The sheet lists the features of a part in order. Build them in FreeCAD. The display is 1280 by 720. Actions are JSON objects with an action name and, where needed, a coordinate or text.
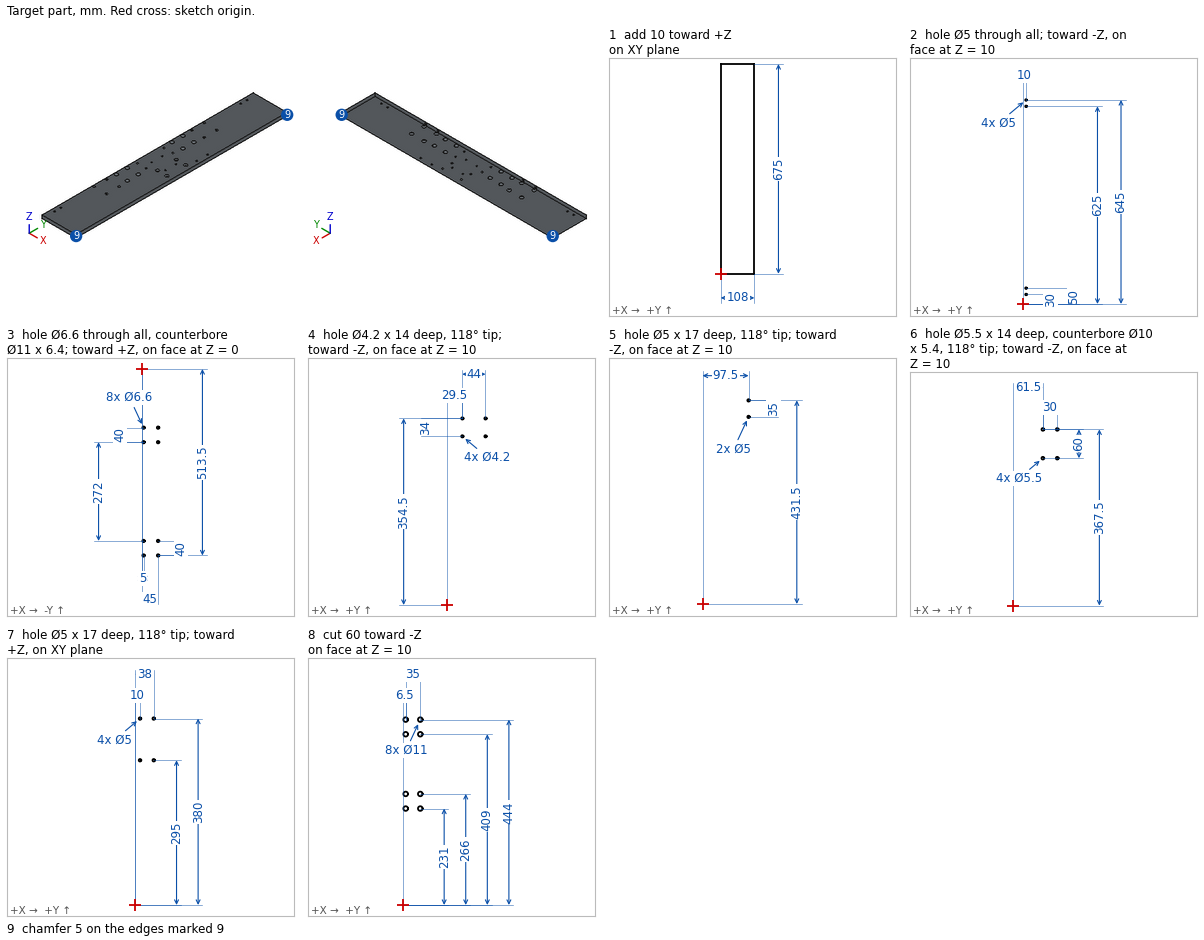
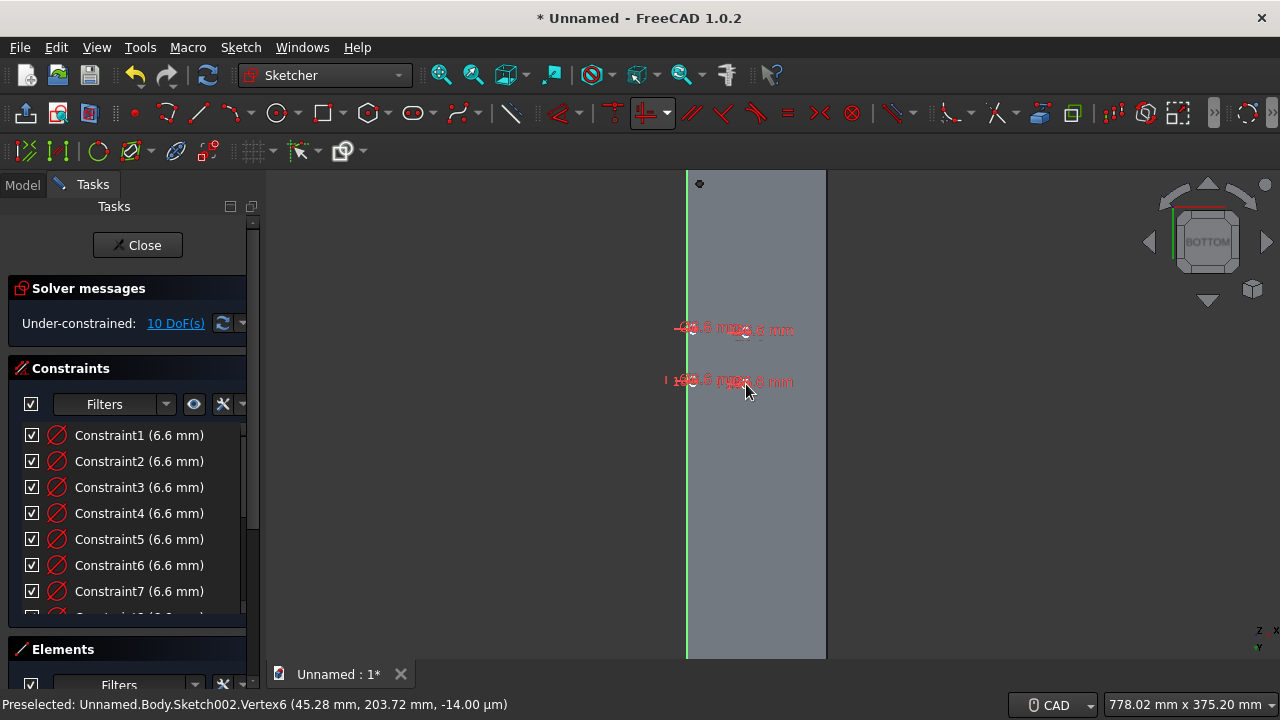
{"action": "left_click", "coordinate": [670, 114]}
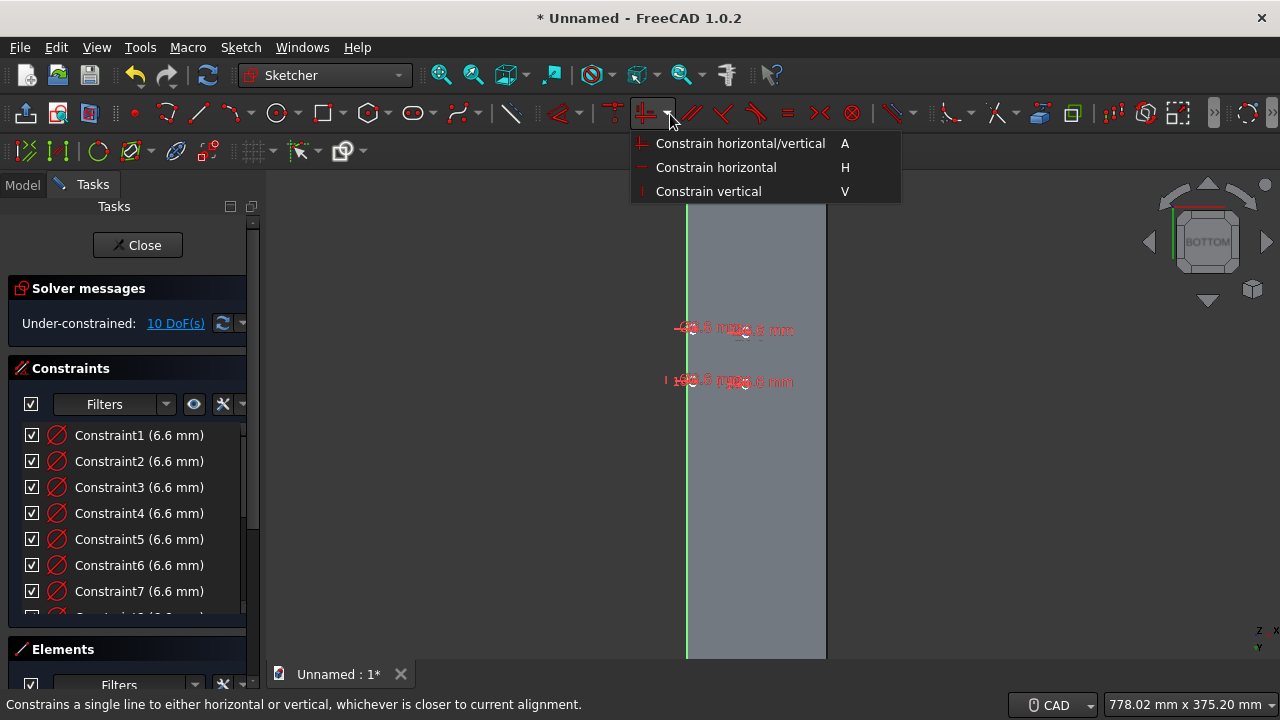
{"action": "left_click", "coordinate": [766, 167]}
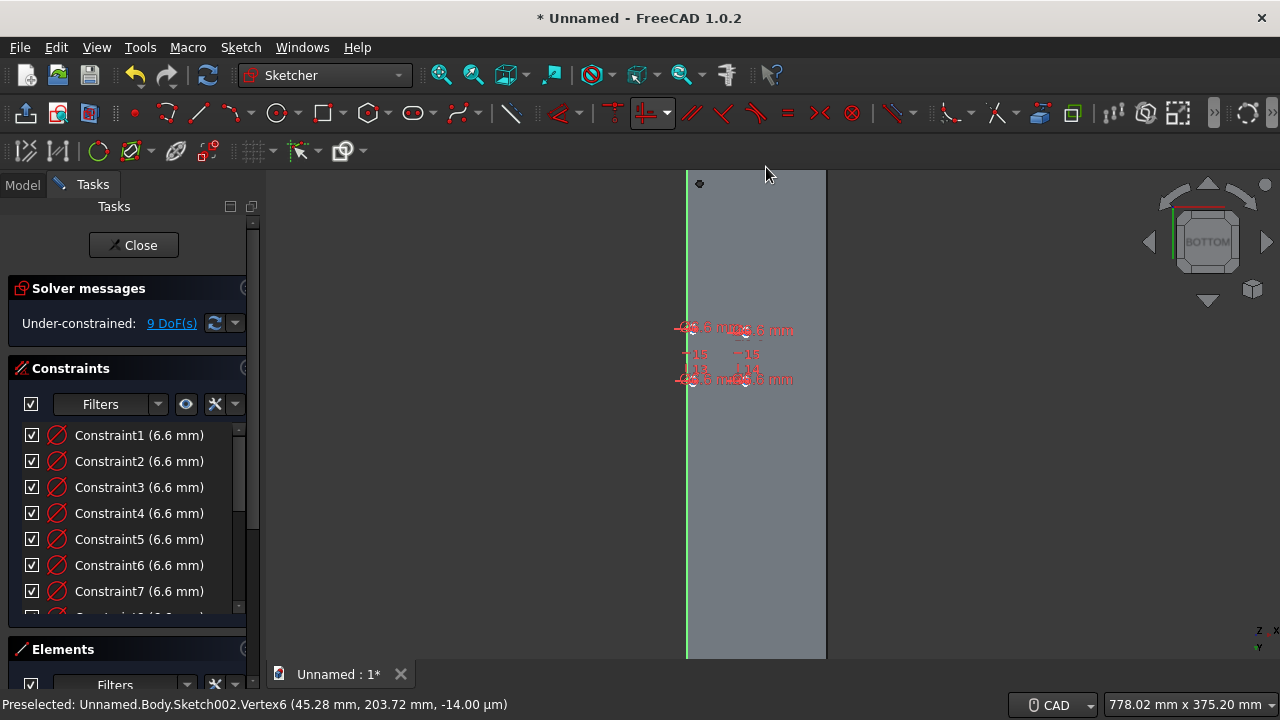
{"action": "left_click", "coordinate": [693, 381]}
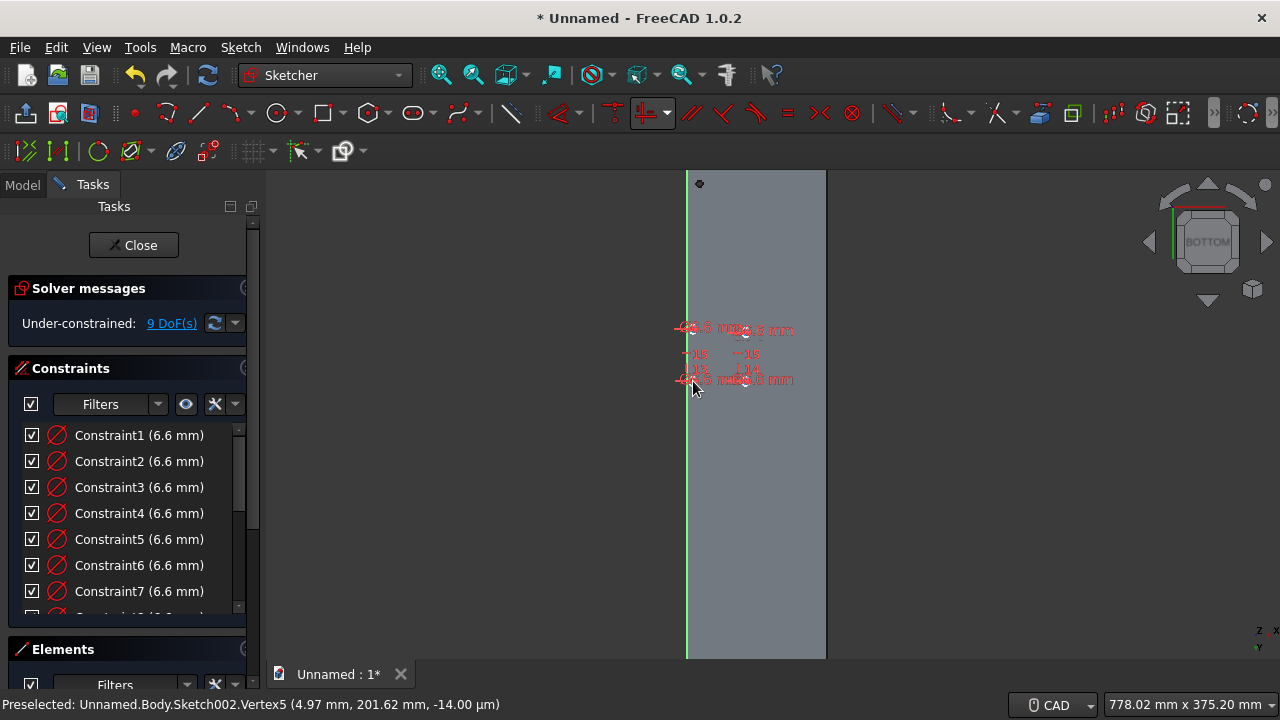
{"action": "left_click", "coordinate": [693, 329]}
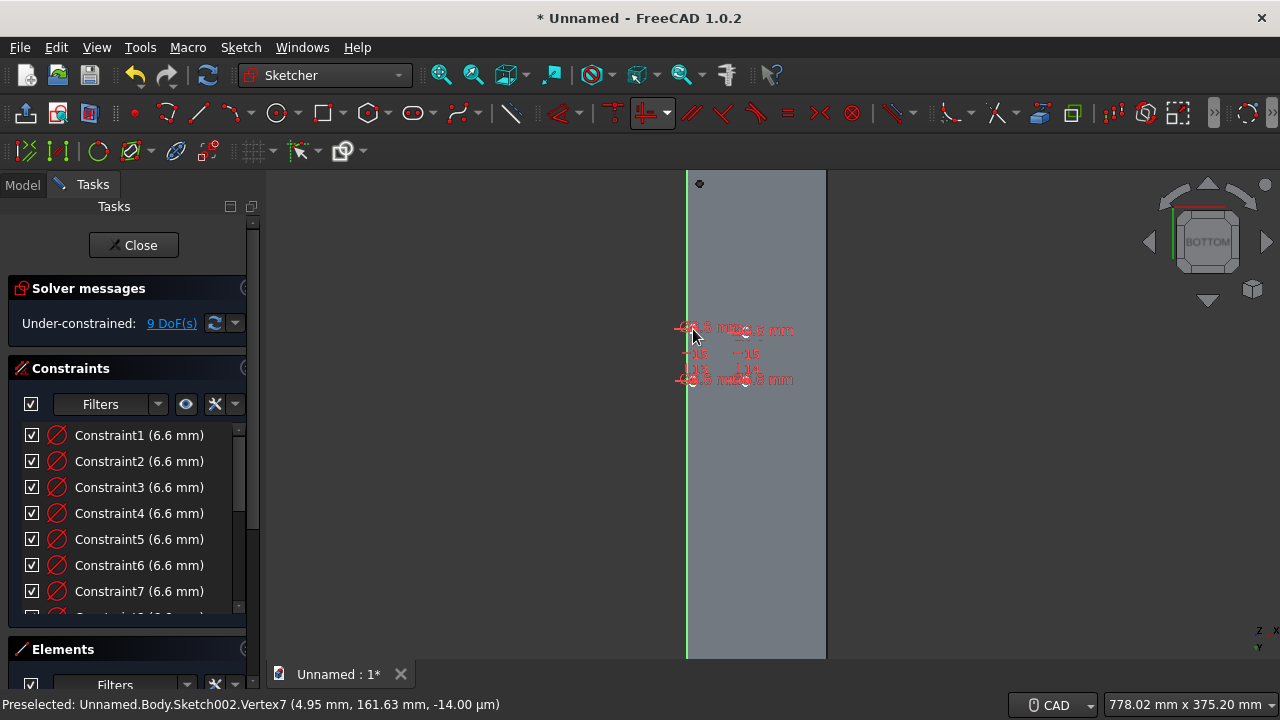
{"action": "left_click", "coordinate": [670, 114]}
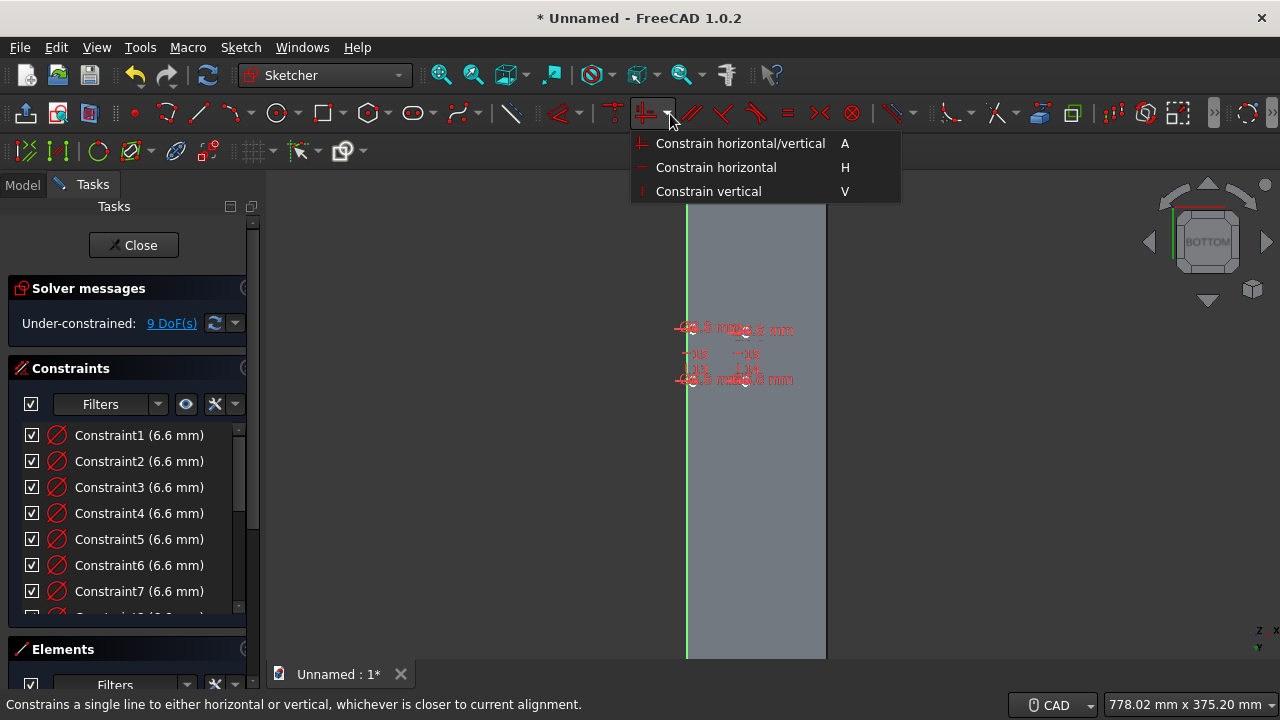
{"action": "left_click", "coordinate": [766, 191]}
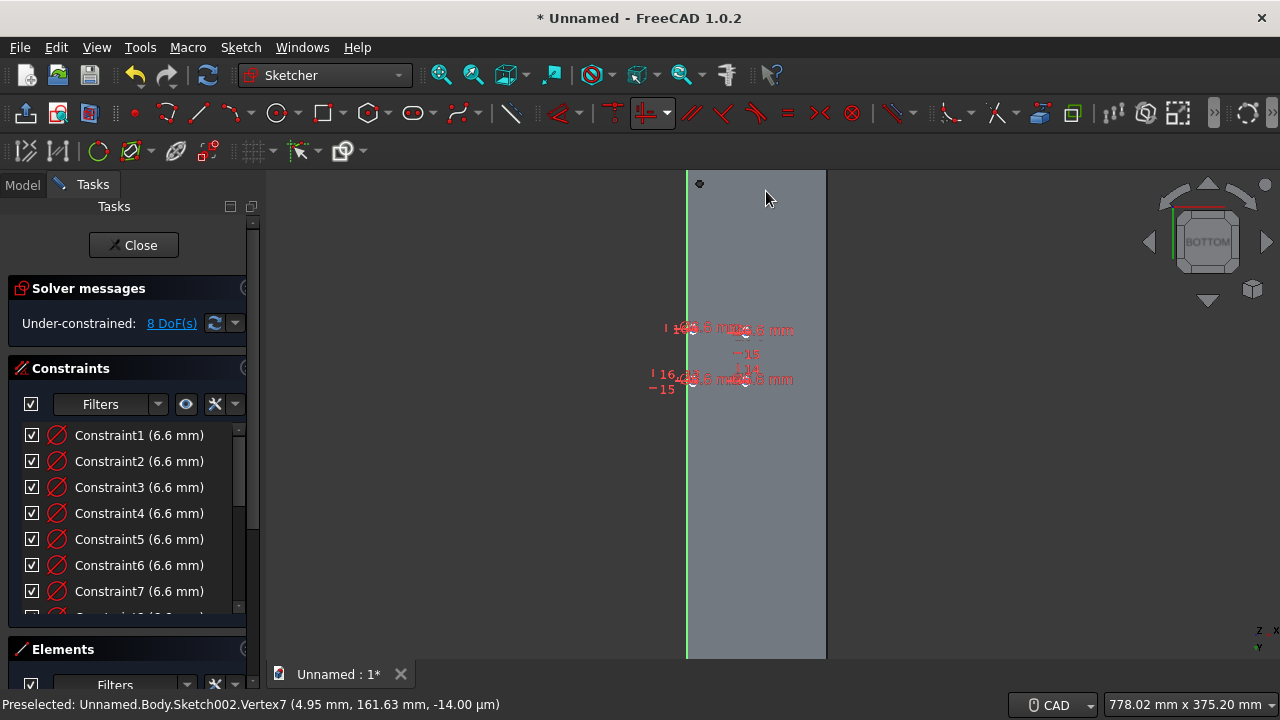
{"action": "left_click", "coordinate": [746, 381]}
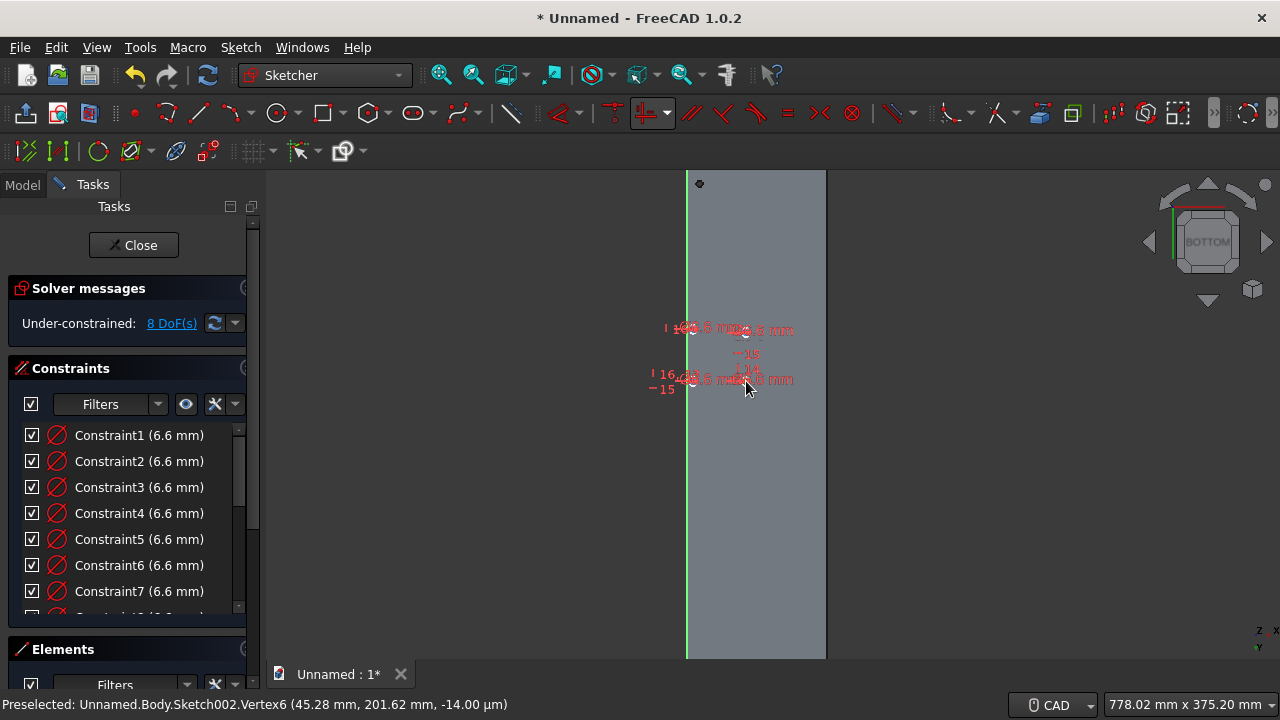
{"action": "left_click", "coordinate": [746, 333]}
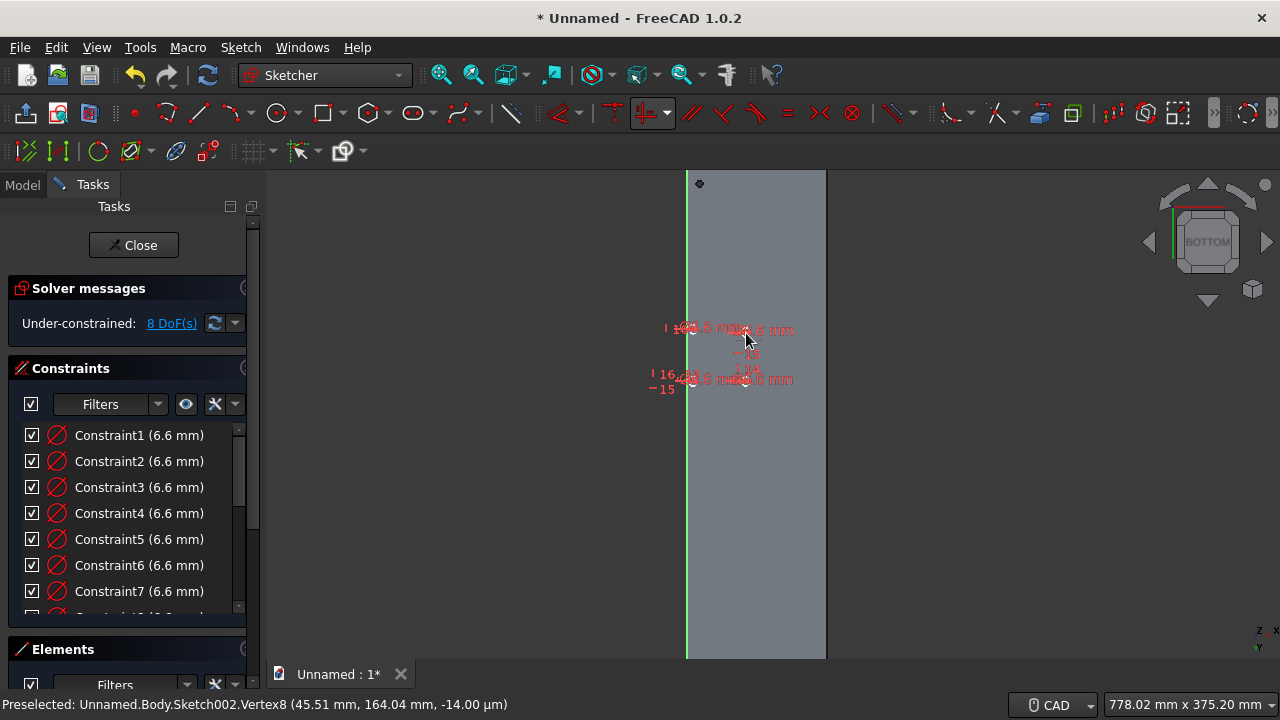
{"action": "left_click", "coordinate": [670, 114]}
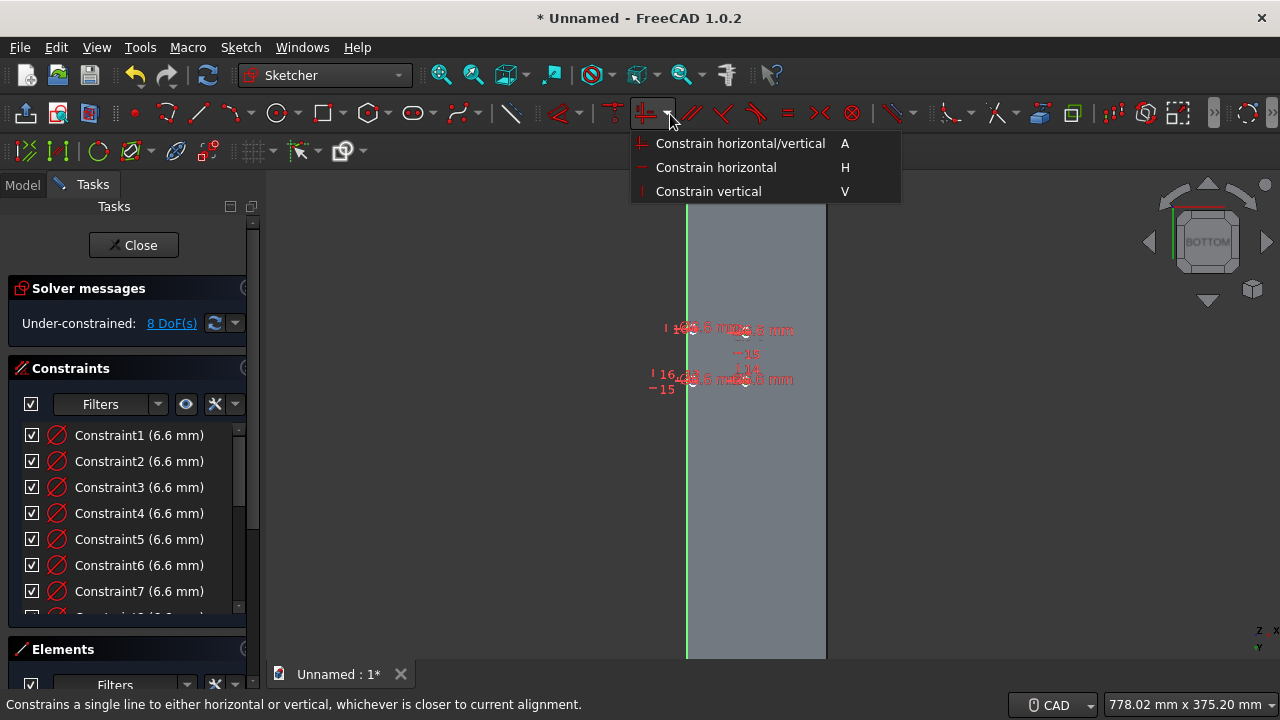
{"action": "left_click", "coordinate": [766, 191]}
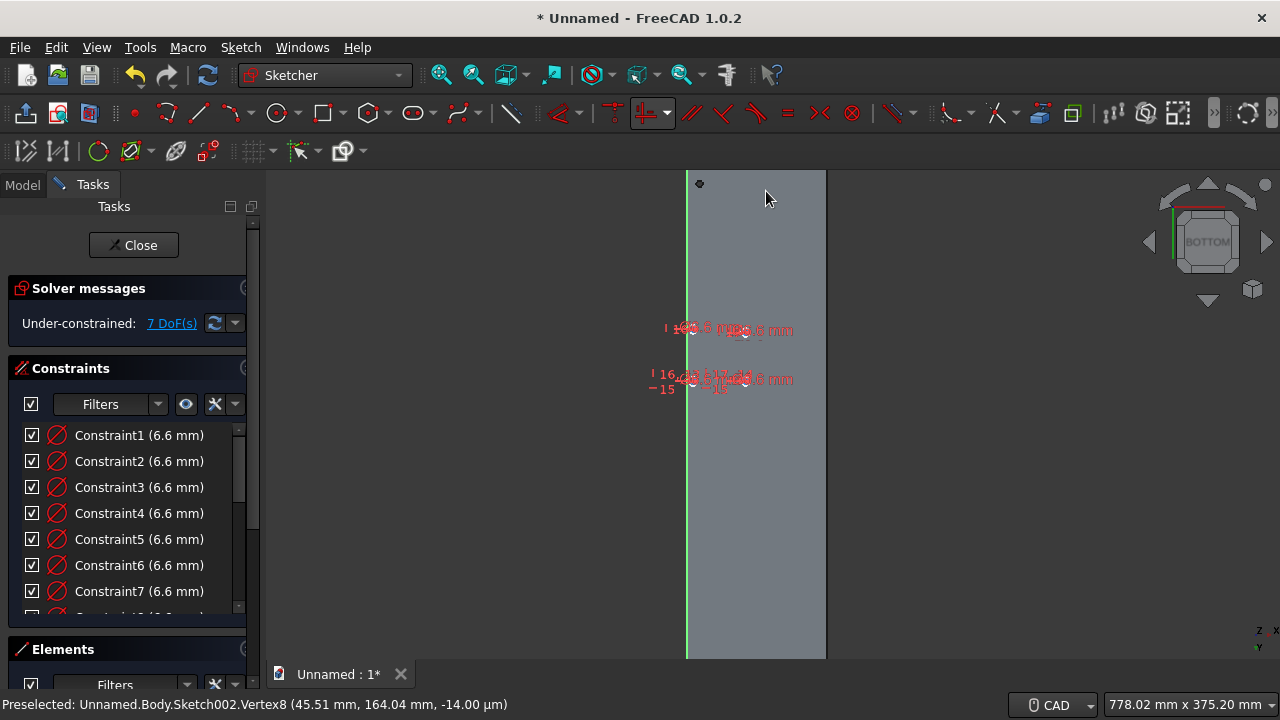
{"action": "left_click", "coordinate": [693, 329]}